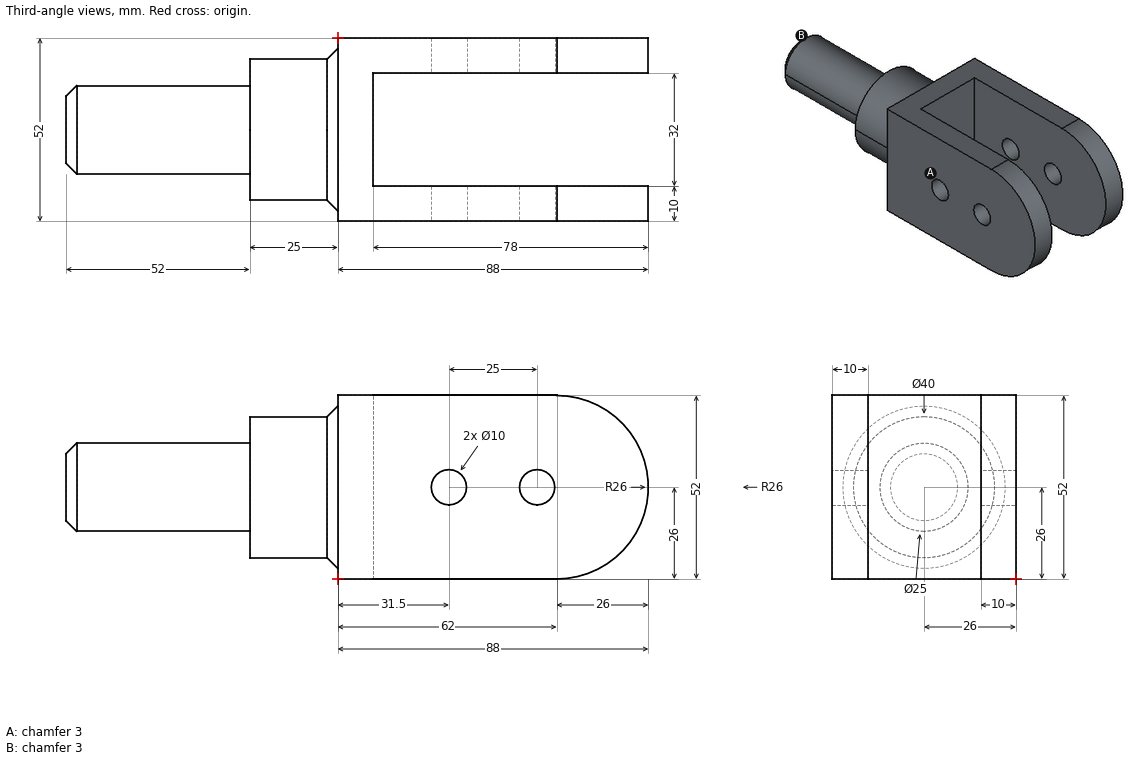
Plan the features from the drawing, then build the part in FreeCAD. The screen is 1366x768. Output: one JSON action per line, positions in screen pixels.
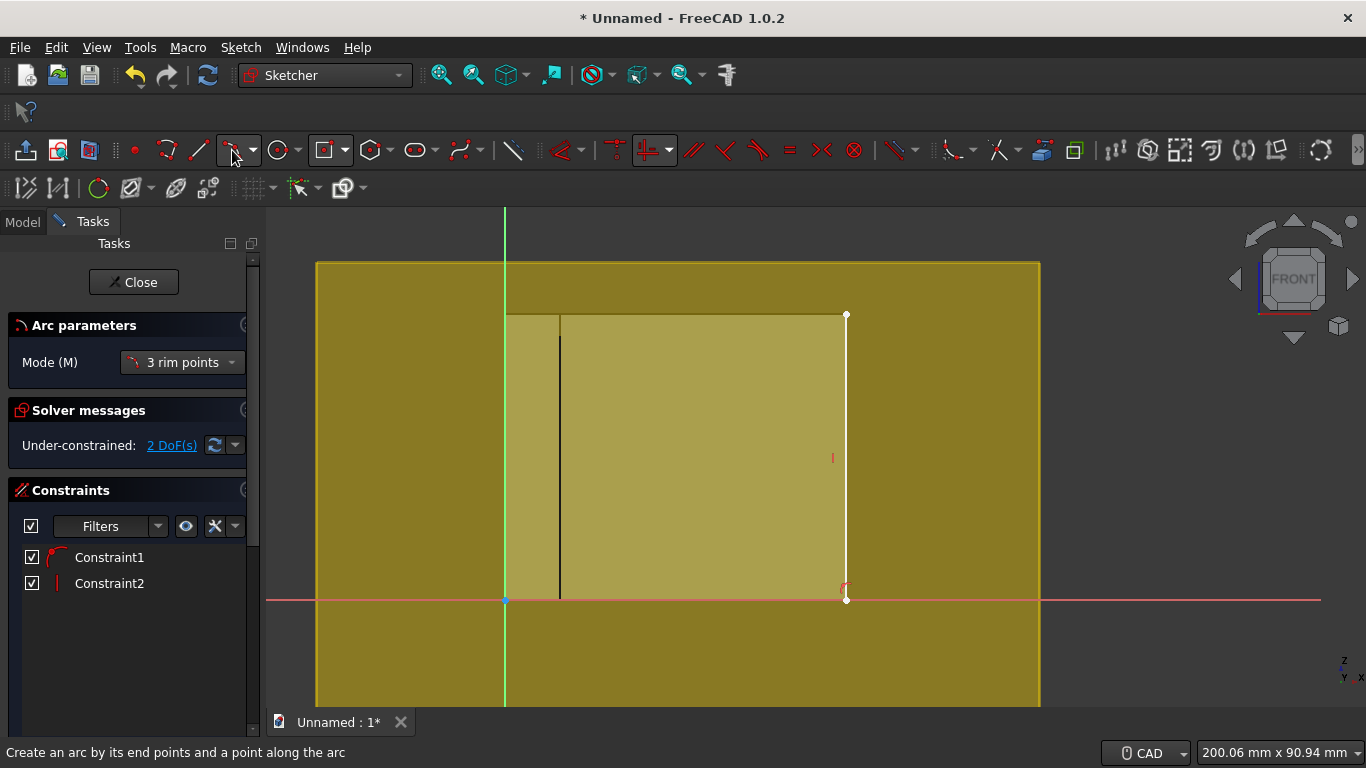
{"action": "left_click", "coordinate": [846, 315]}
{"action": "left_click", "coordinate": [846, 600]}
{"action": "left_click", "coordinate": [989, 457]}
{"action": "key", "text": "Escape"}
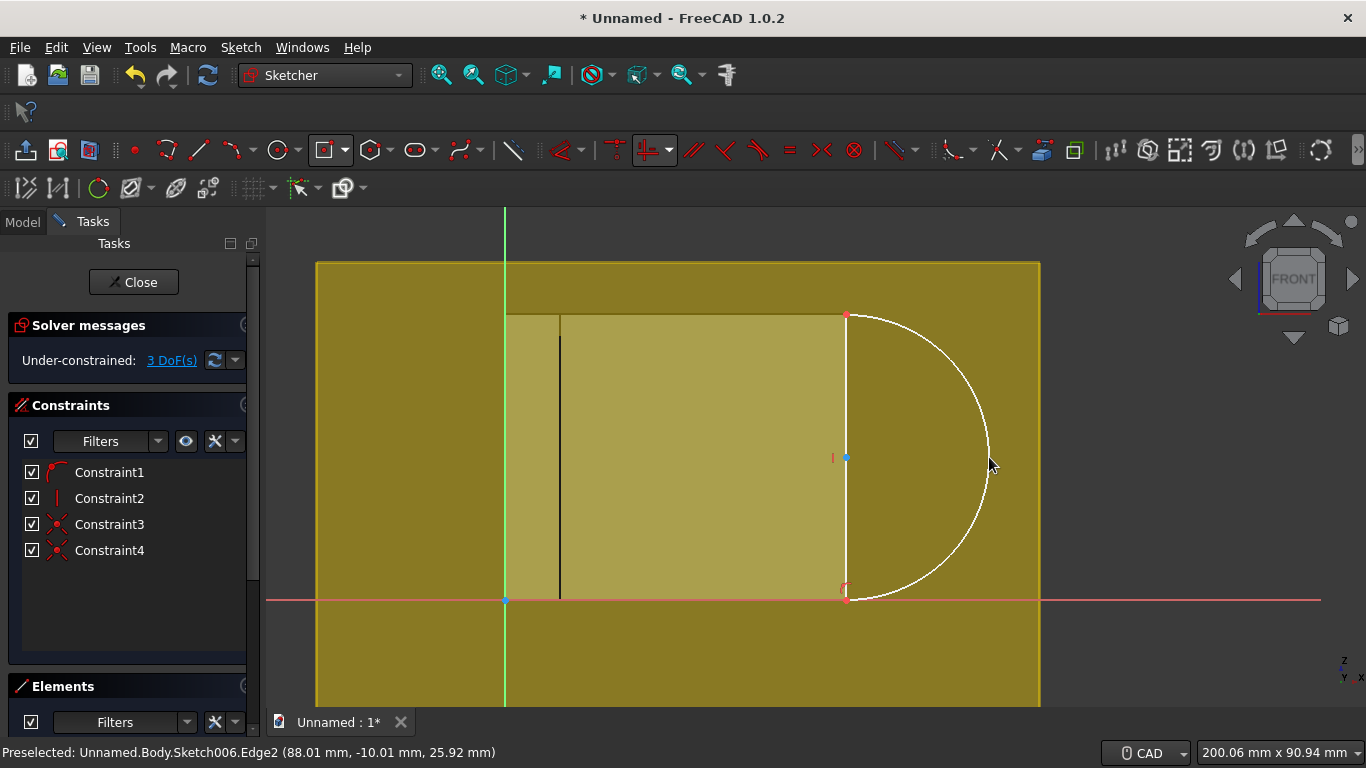
{"action": "left_click", "coordinate": [560, 150]}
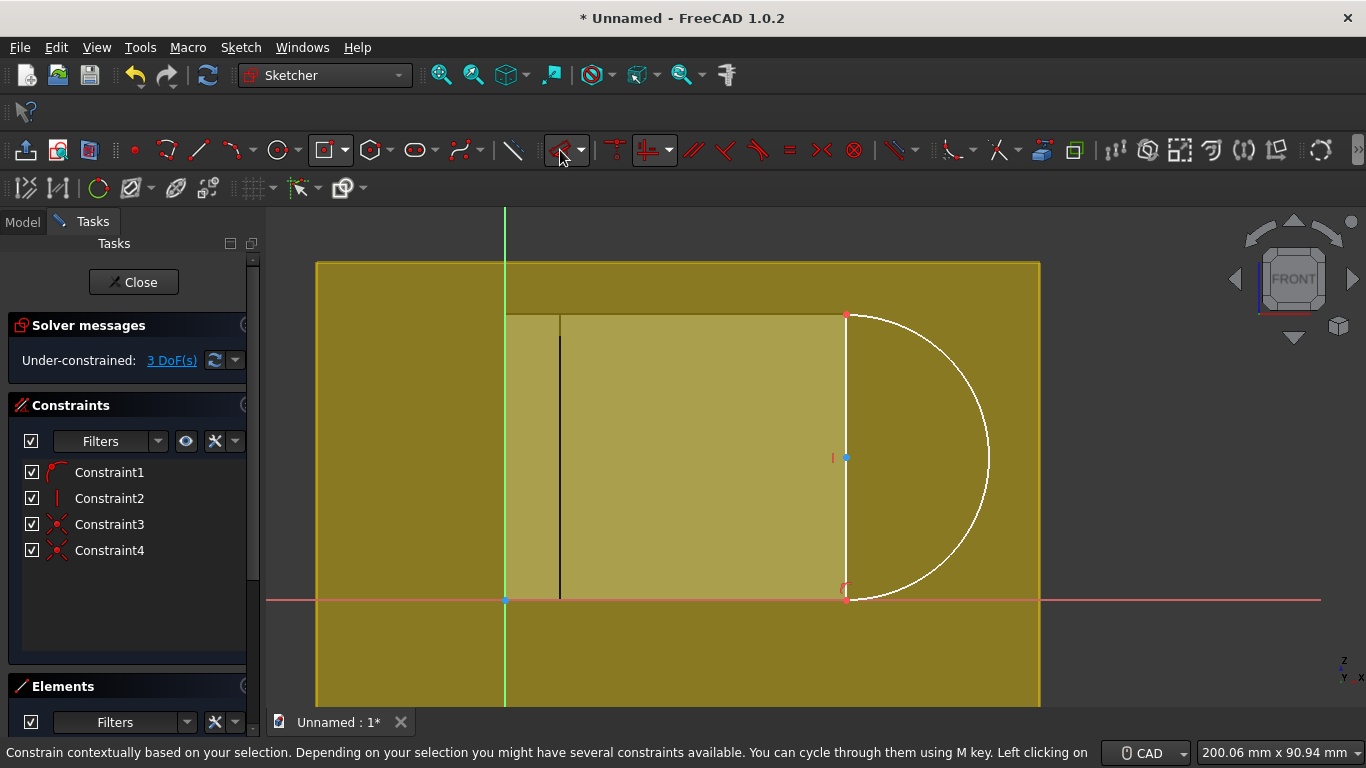
{"action": "left_click", "coordinate": [962, 541]}
{"action": "left_click", "coordinate": [988, 560]}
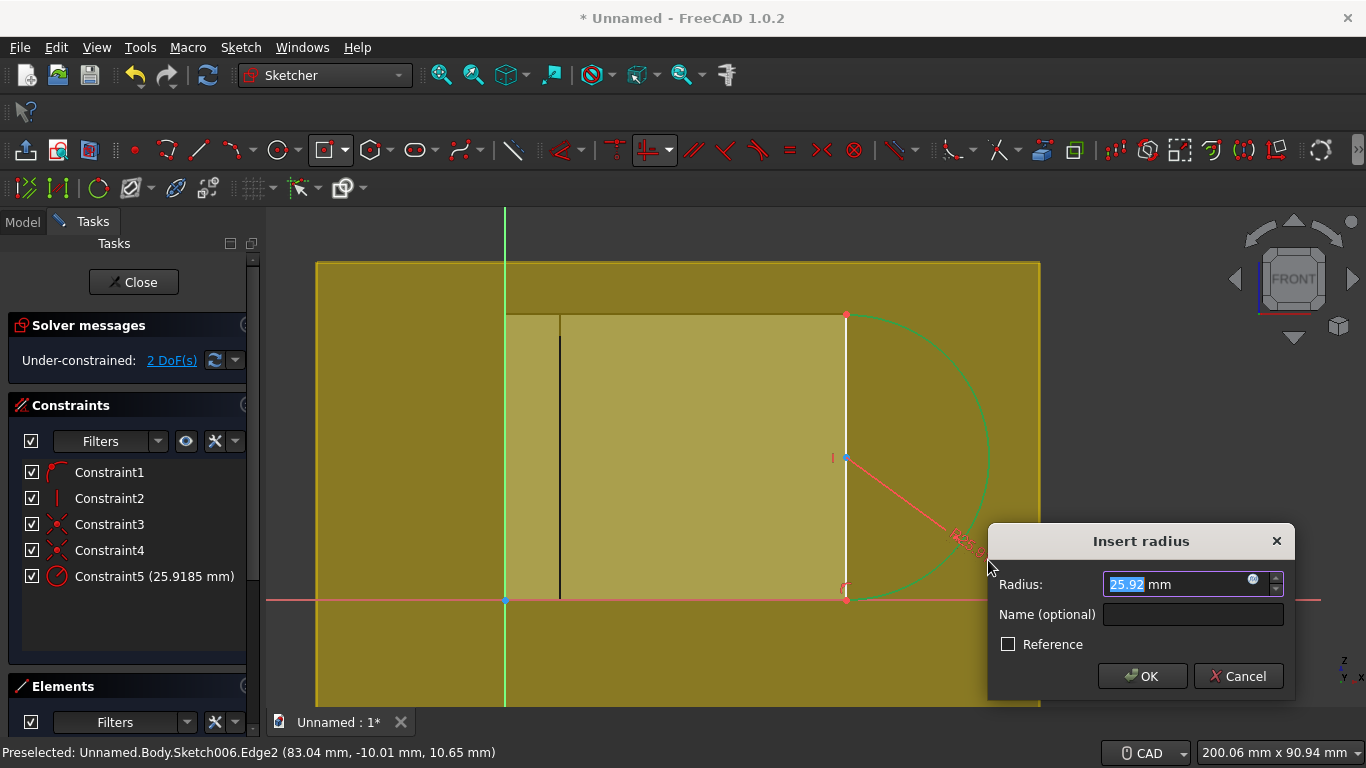
{"action": "type", "text": "26"}
{"action": "key", "text": "Return"}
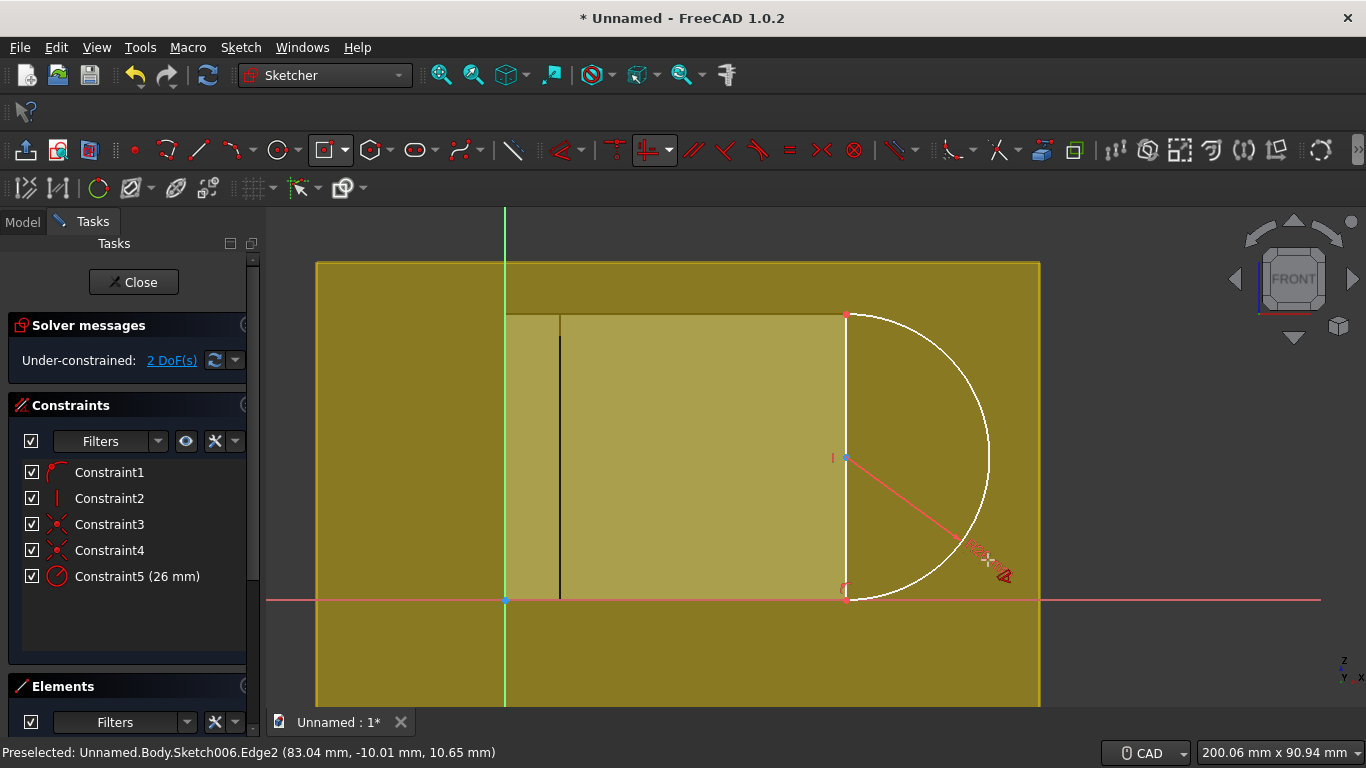
{"action": "left_click", "coordinate": [846, 600]}
{"action": "left_click", "coordinate": [676, 634]}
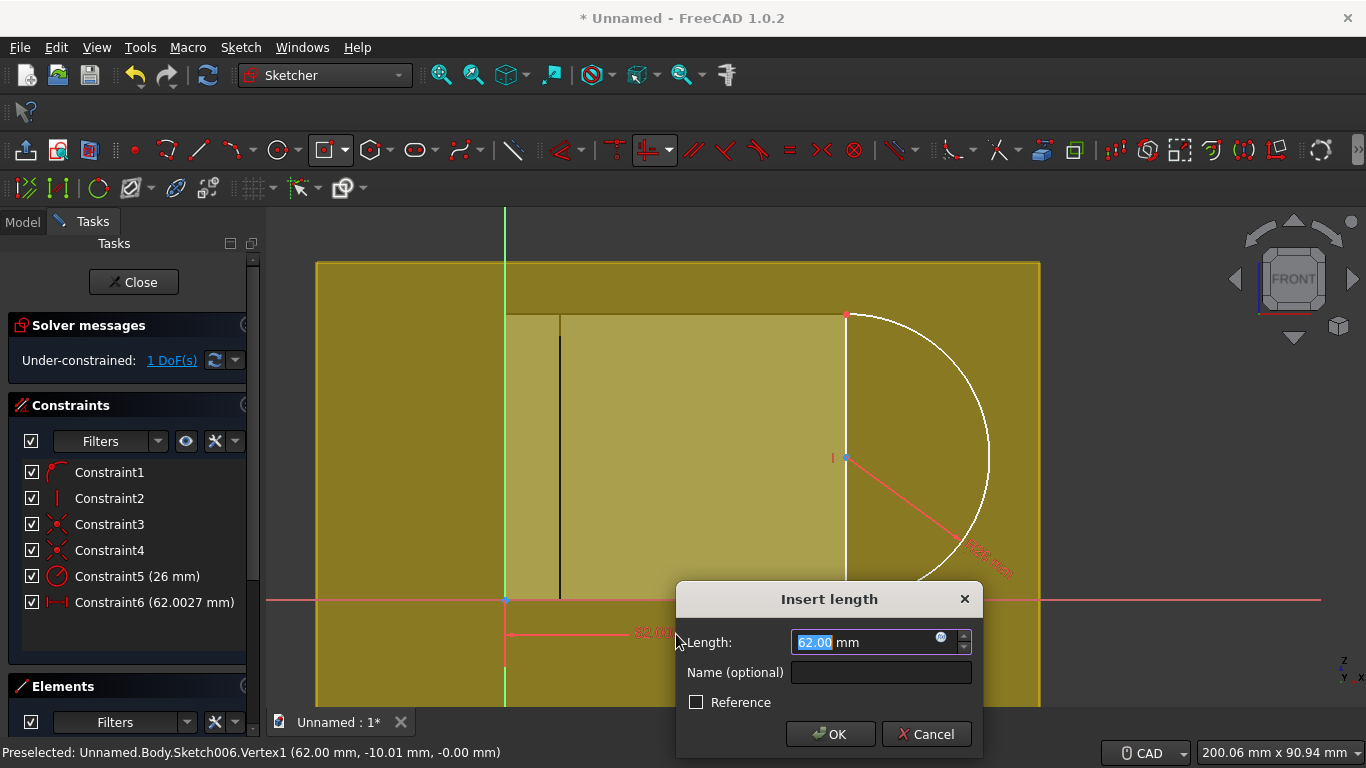
{"action": "type", "text": "62"}
{"action": "key", "text": "Return"}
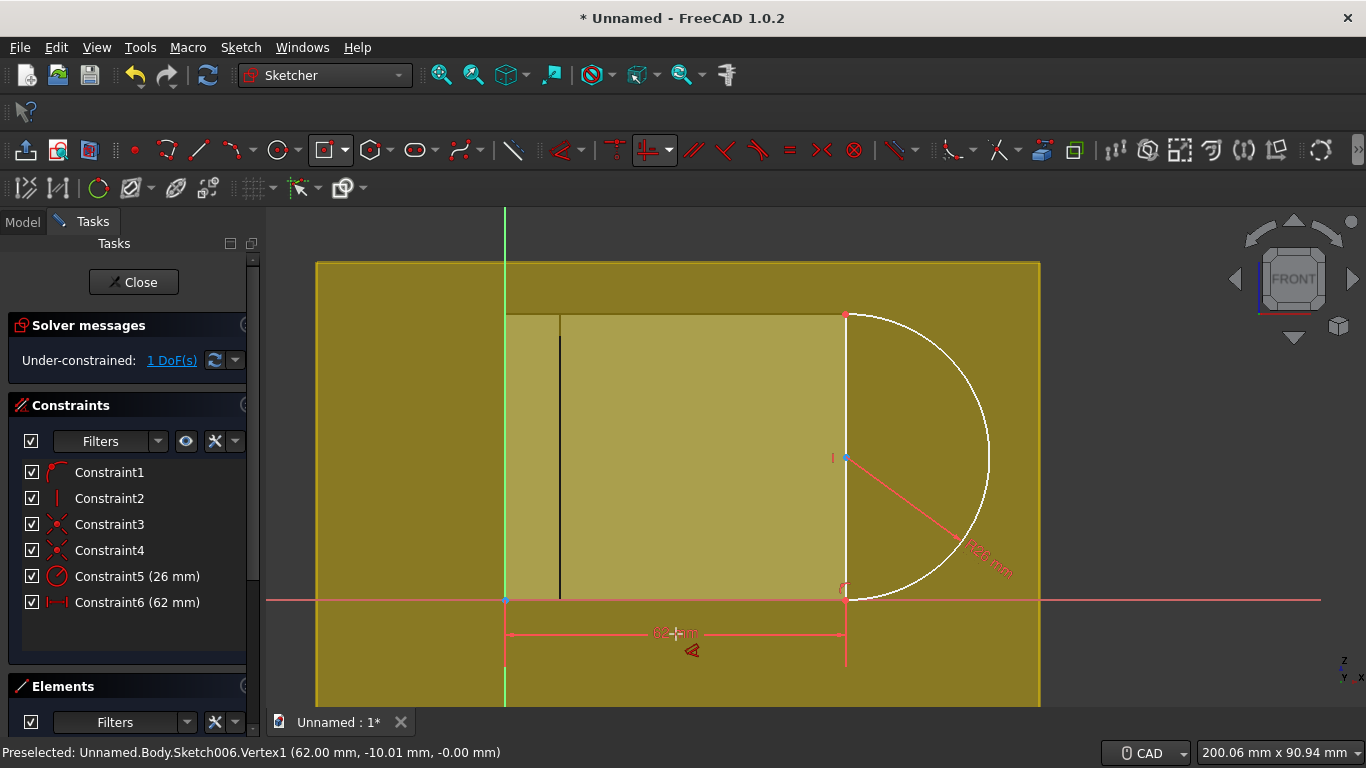
{"action": "left_click", "coordinate": [846, 457]}
{"action": "left_click", "coordinate": [597, 634]}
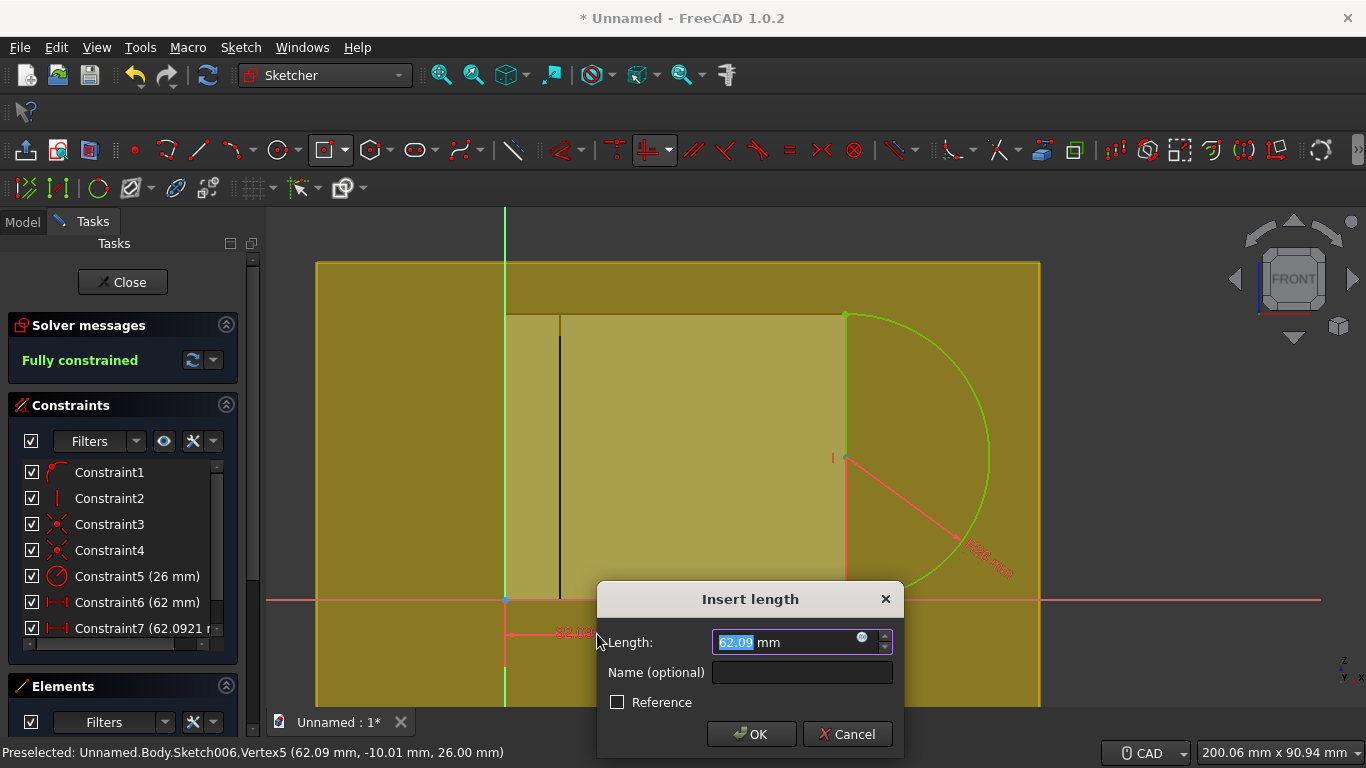
{"action": "type", "text": "62"}
{"action": "key", "text": "Return"}
{"action": "key", "text": "Escape"}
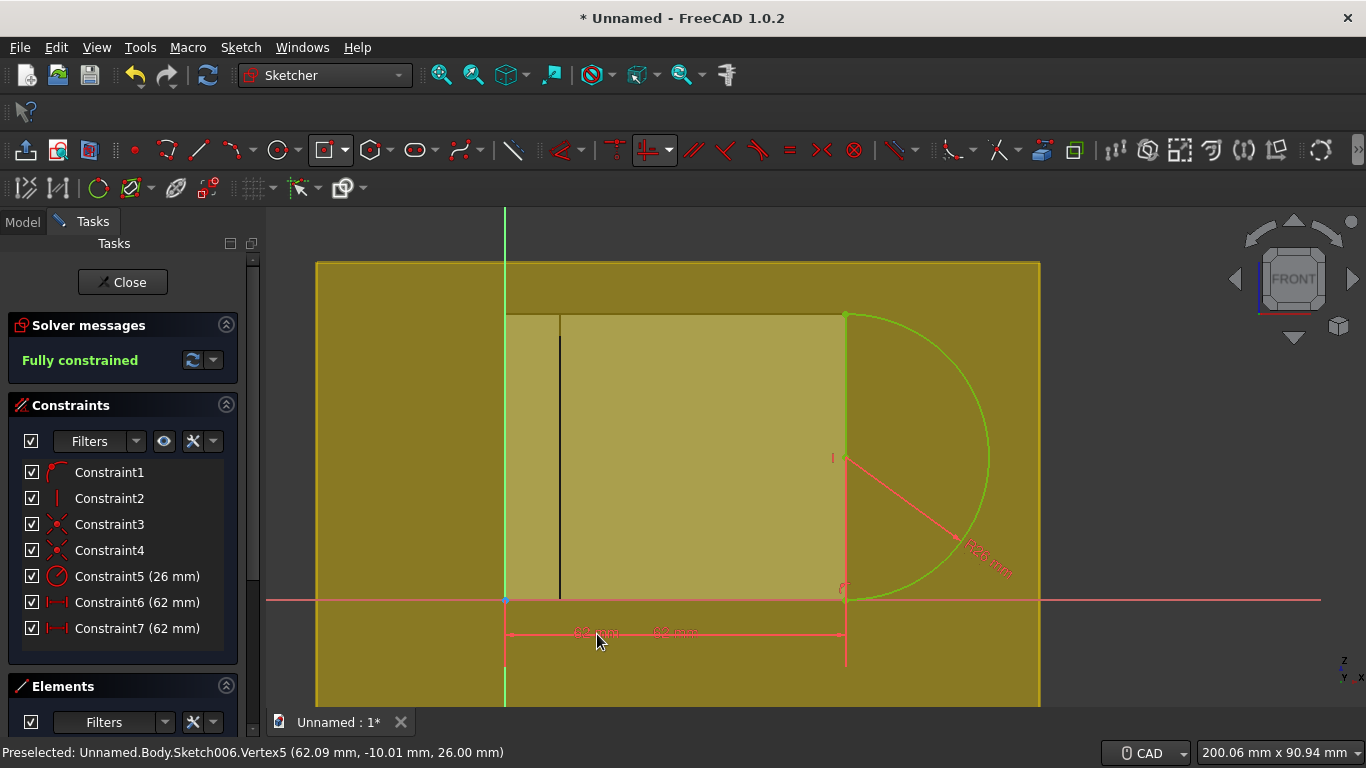
{"action": "left_click", "coordinate": [123, 282]}